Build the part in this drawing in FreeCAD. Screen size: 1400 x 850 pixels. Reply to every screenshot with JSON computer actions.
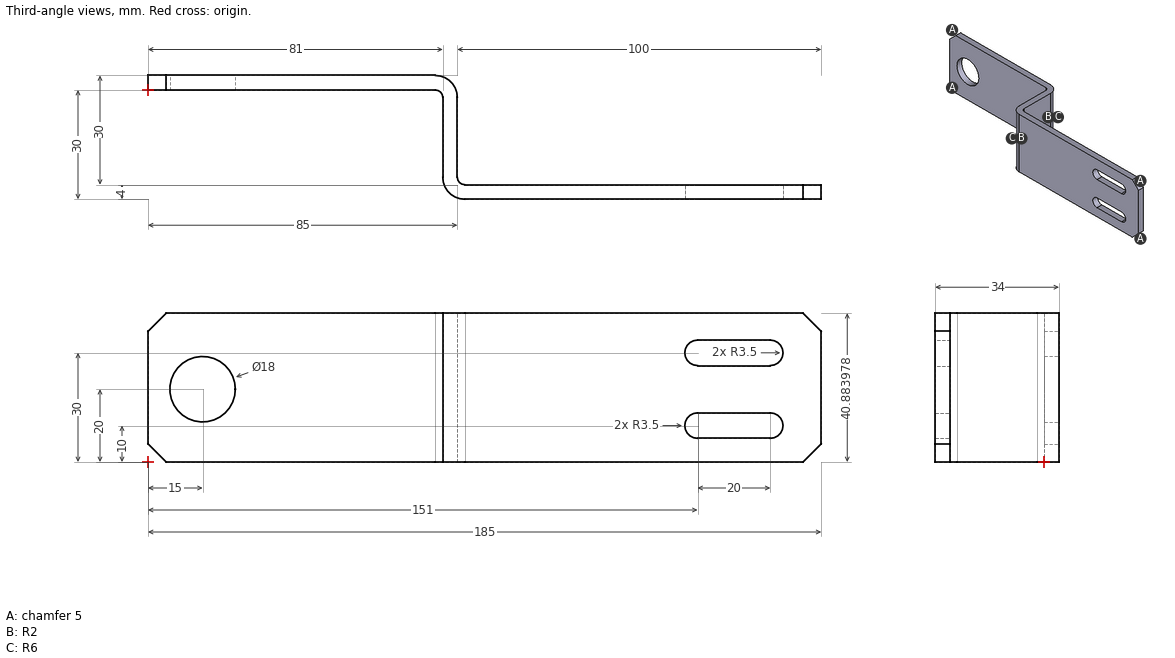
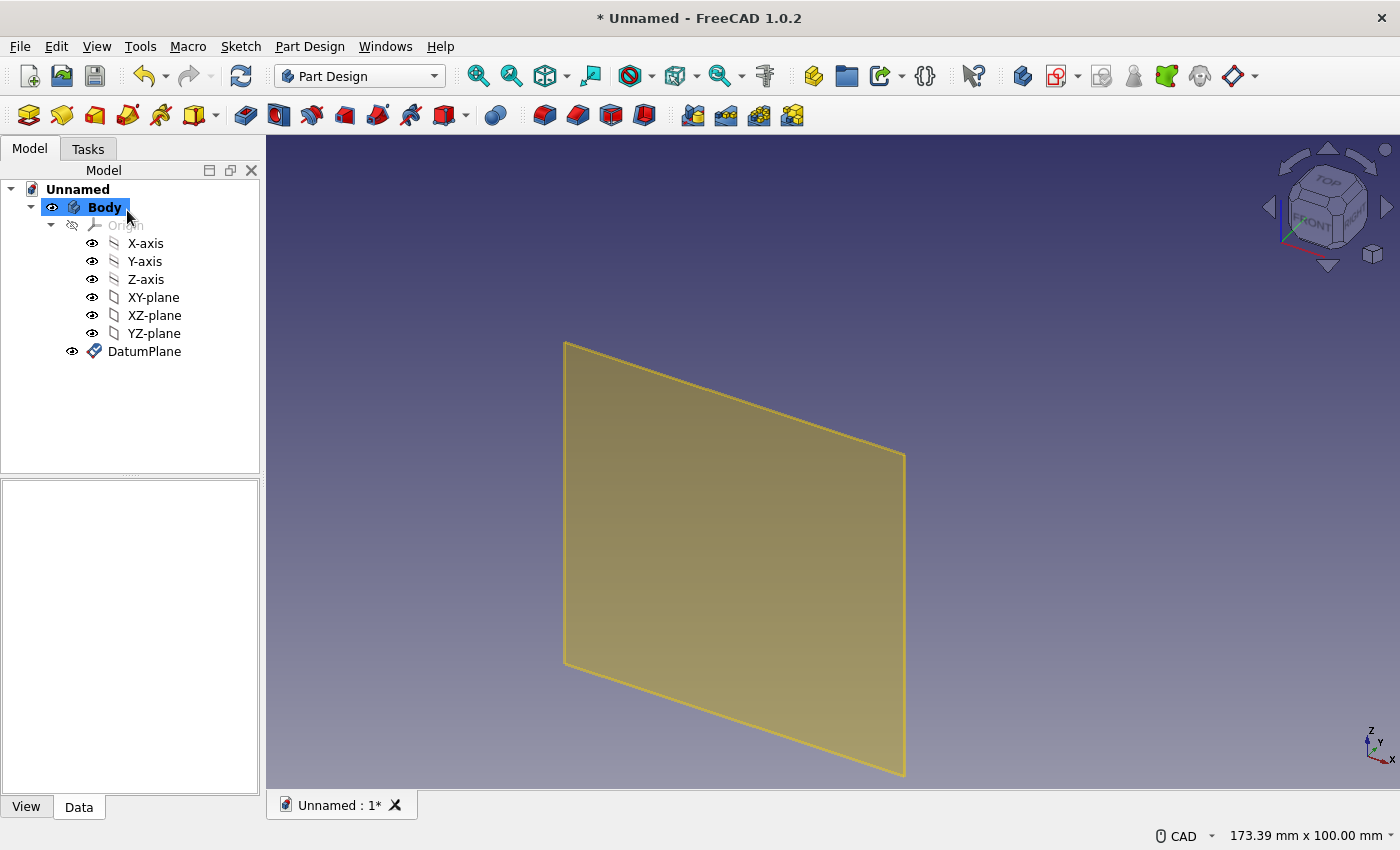
{"action": "left_click", "coordinate": [117, 351]}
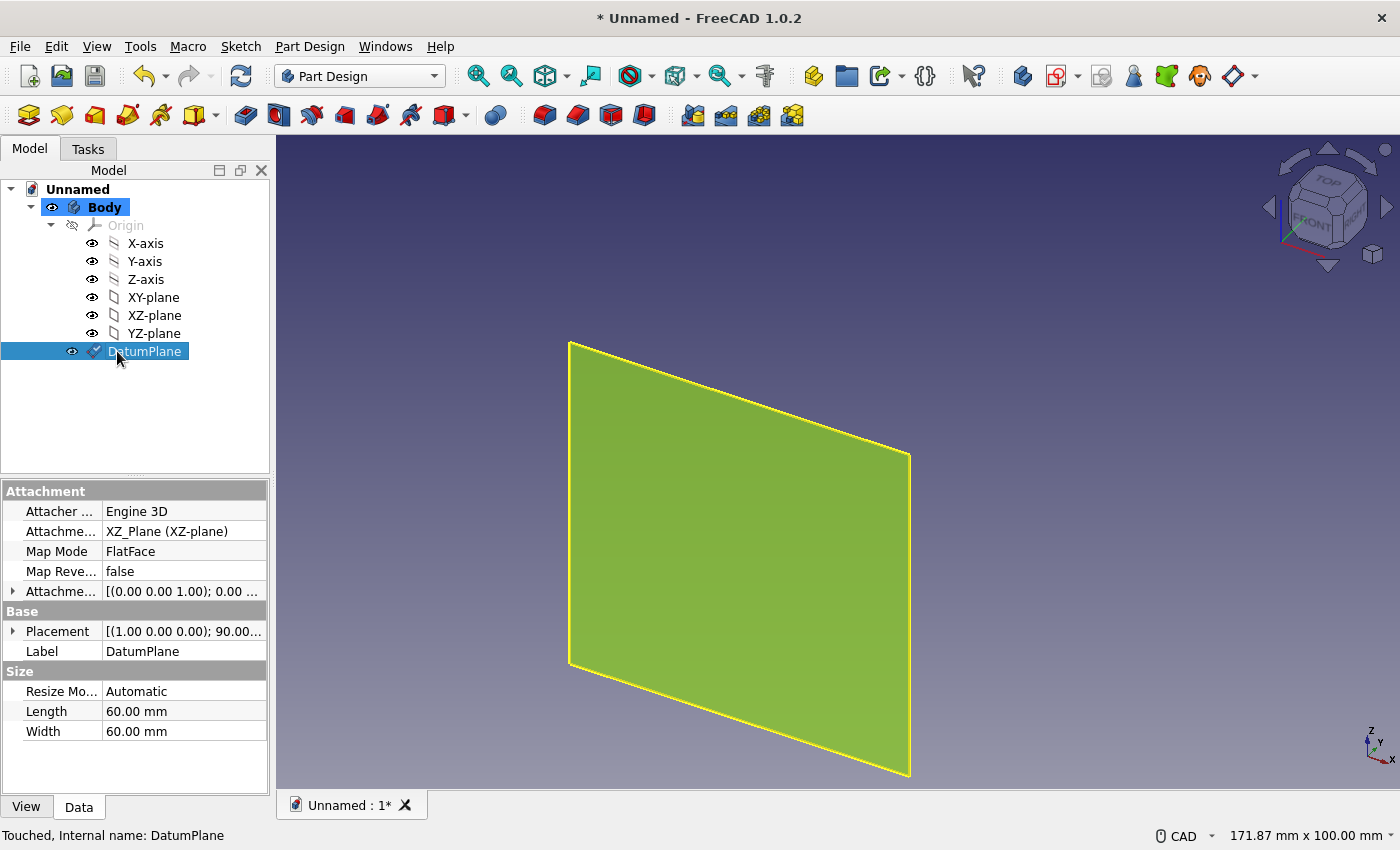
{"action": "left_click", "coordinate": [1056, 76]}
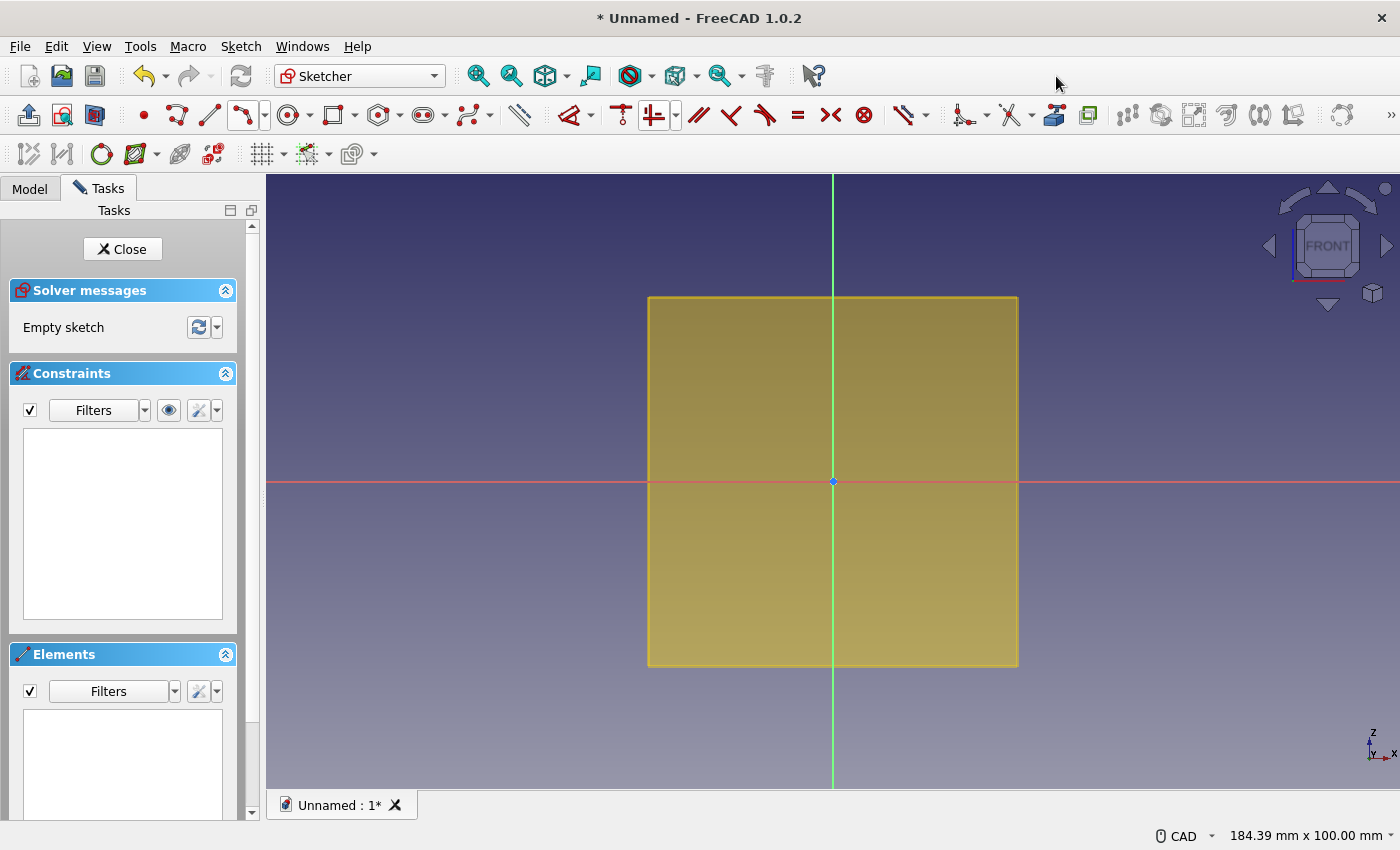
{"action": "scroll", "coordinate": [294, 584], "scroll_direction": "down", "scroll_amount": 4}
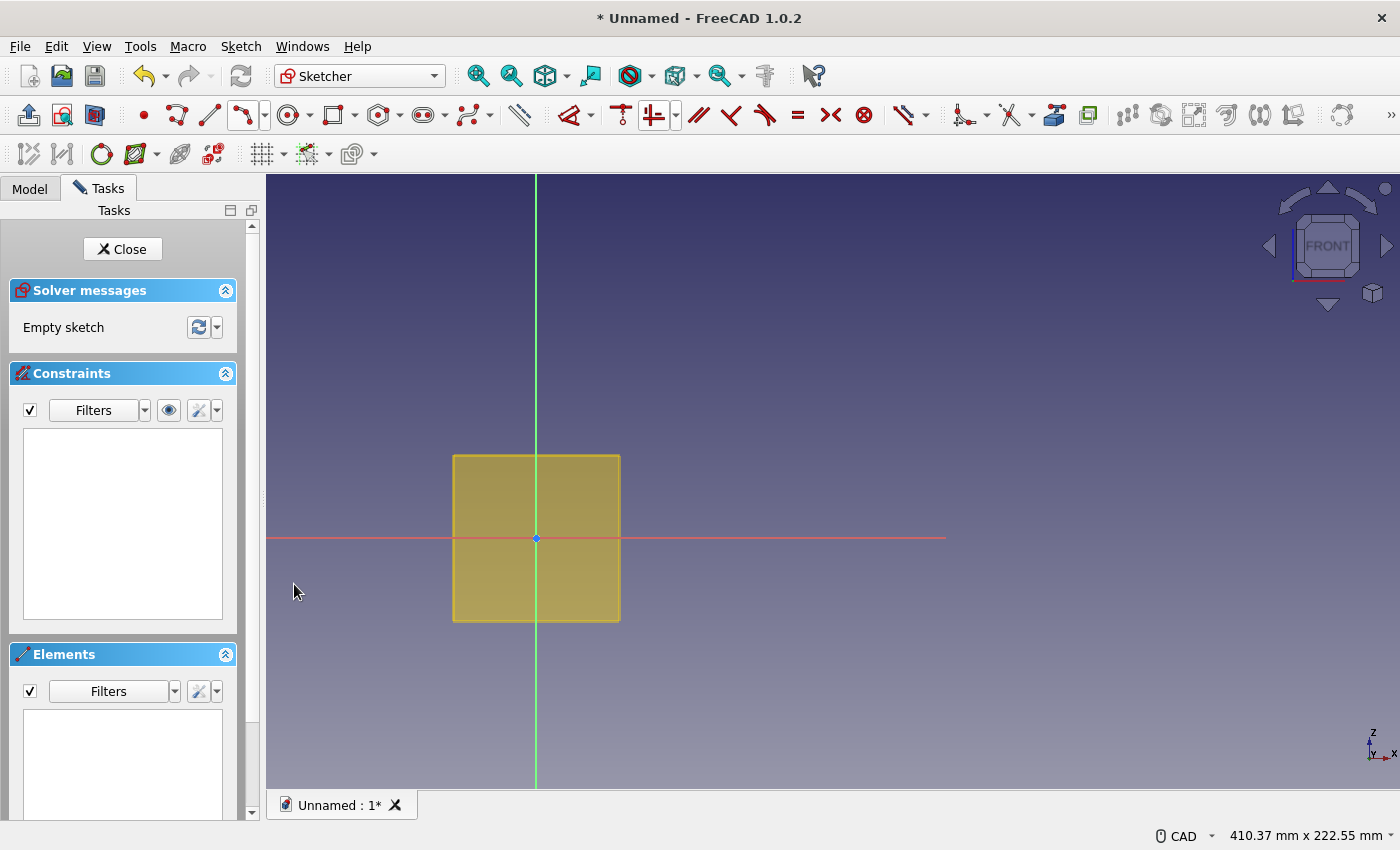
{"action": "left_click", "coordinate": [332, 116]}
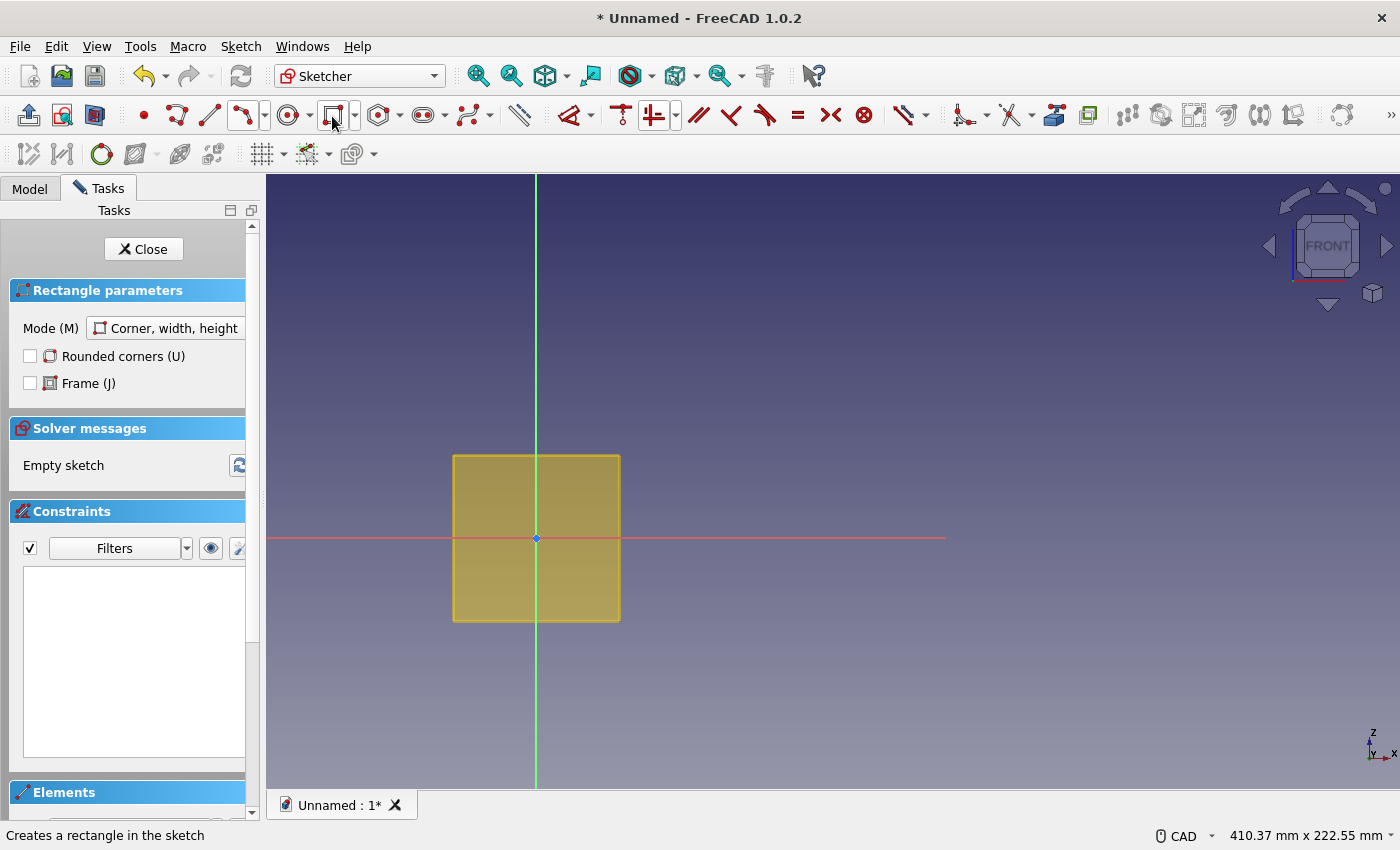
{"action": "left_click", "coordinate": [536, 538]}
{"action": "left_click", "coordinate": [1047, 425]}
{"action": "key", "text": "Escape"}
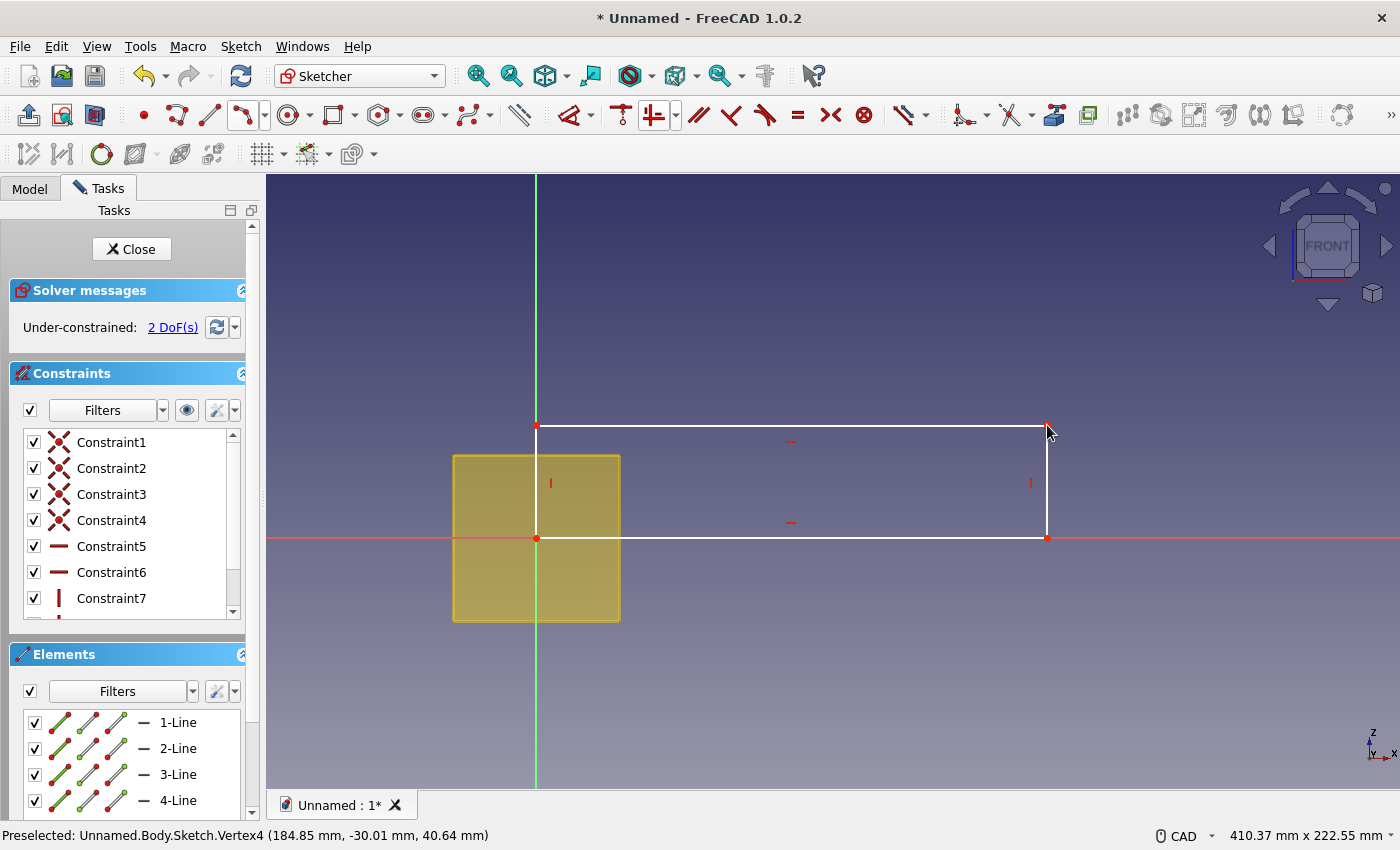
{"action": "left_click", "coordinate": [568, 116]}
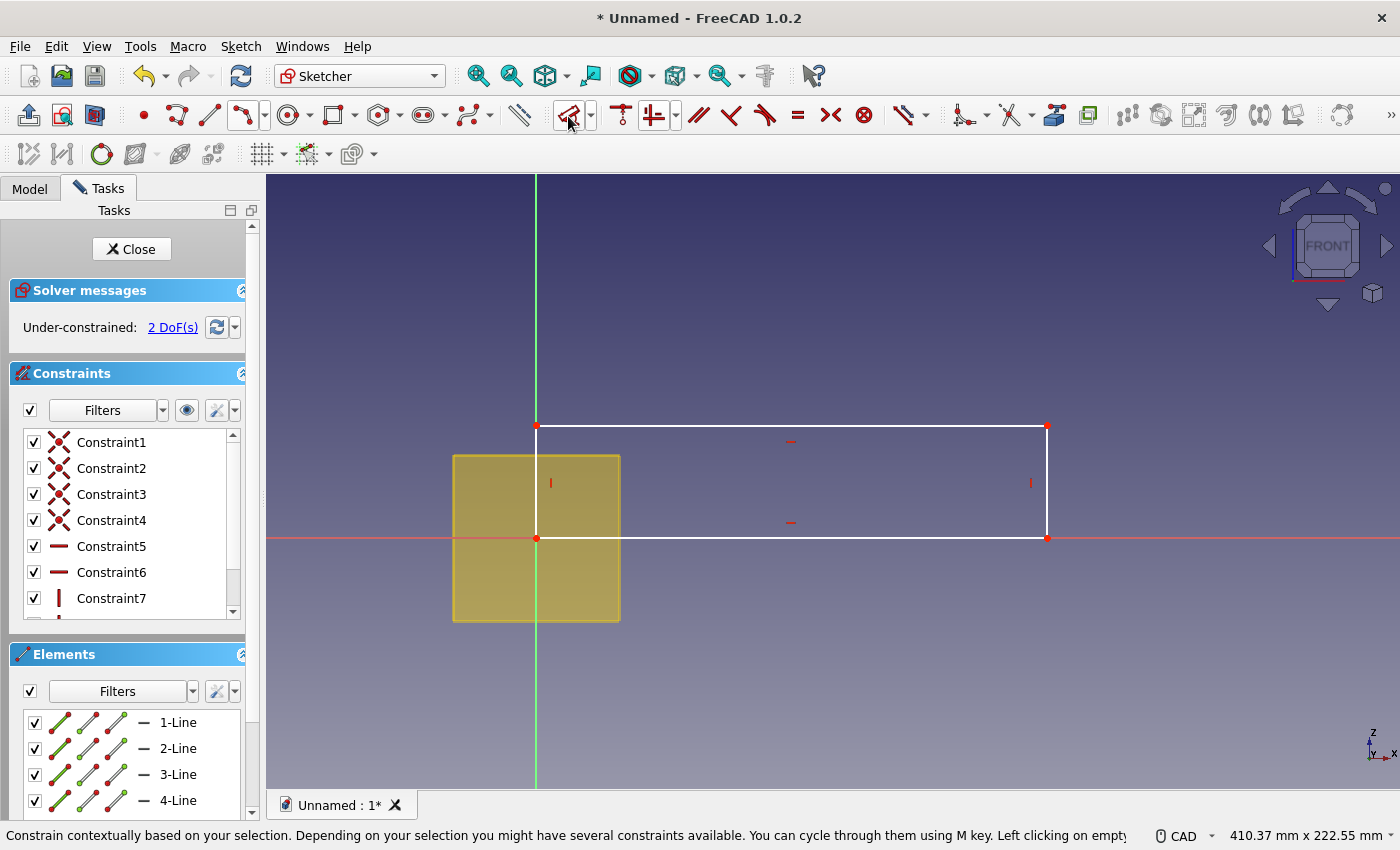
{"action": "left_click", "coordinate": [689, 538]}
{"action": "left_click", "coordinate": [792, 572]}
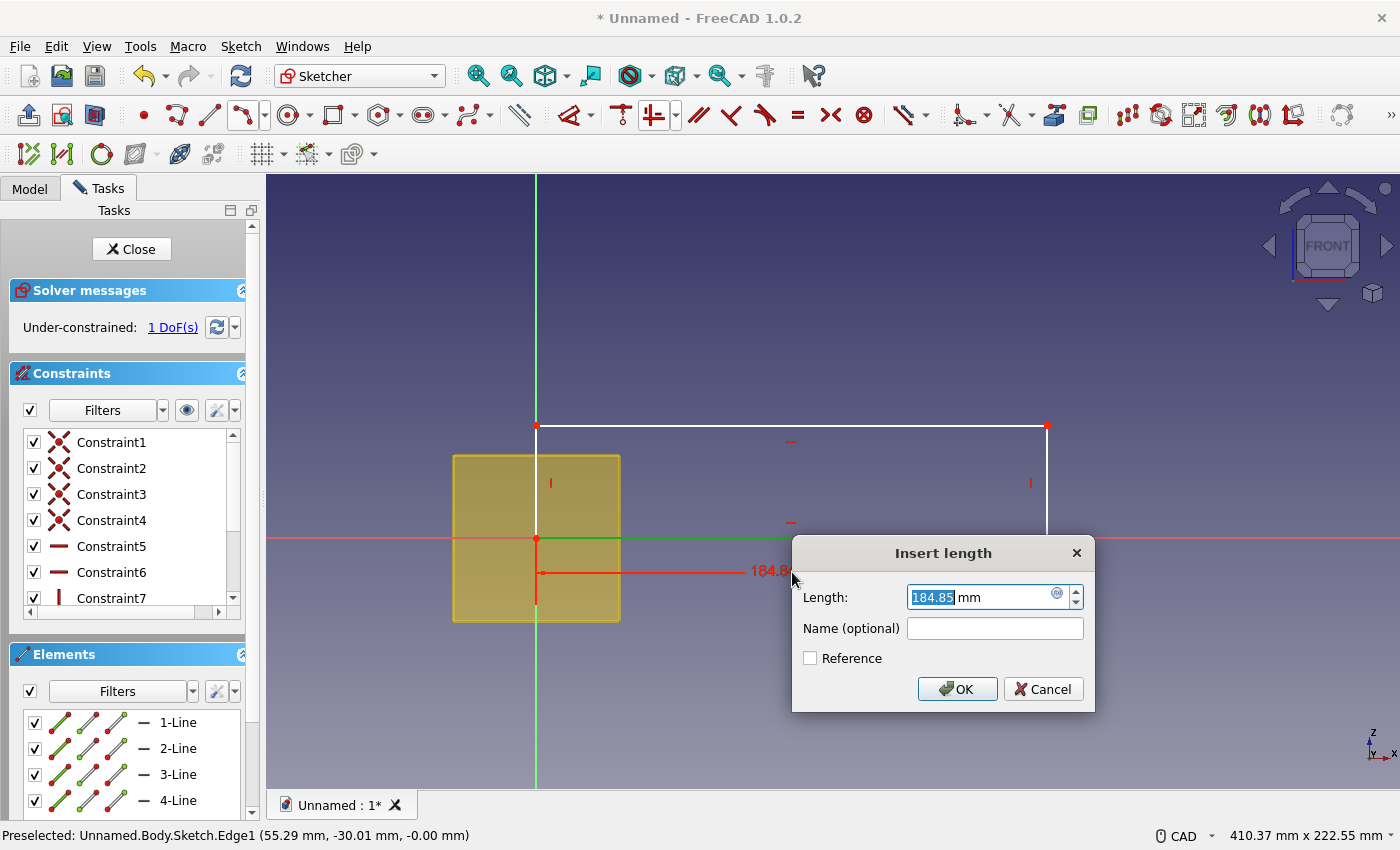
{"action": "type", "text": "185"}
{"action": "key", "text": "Return"}